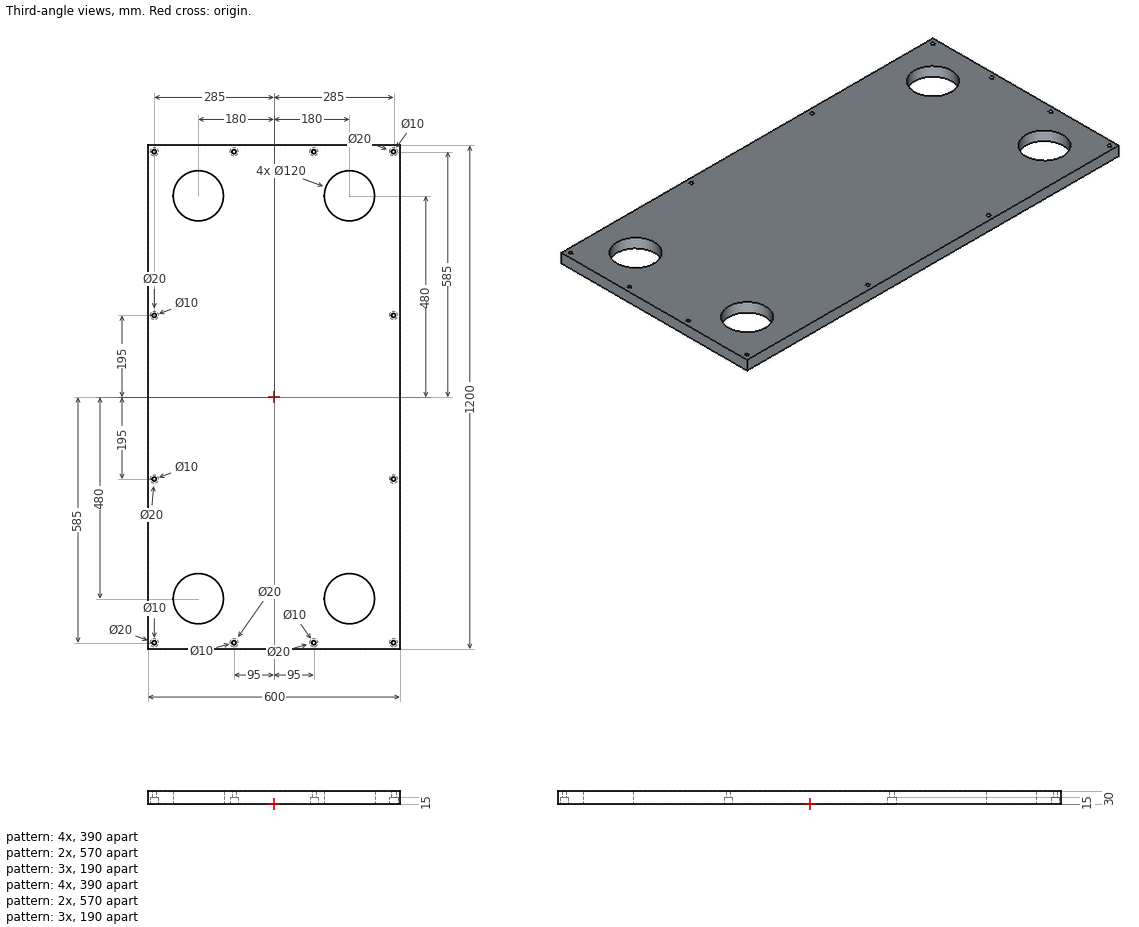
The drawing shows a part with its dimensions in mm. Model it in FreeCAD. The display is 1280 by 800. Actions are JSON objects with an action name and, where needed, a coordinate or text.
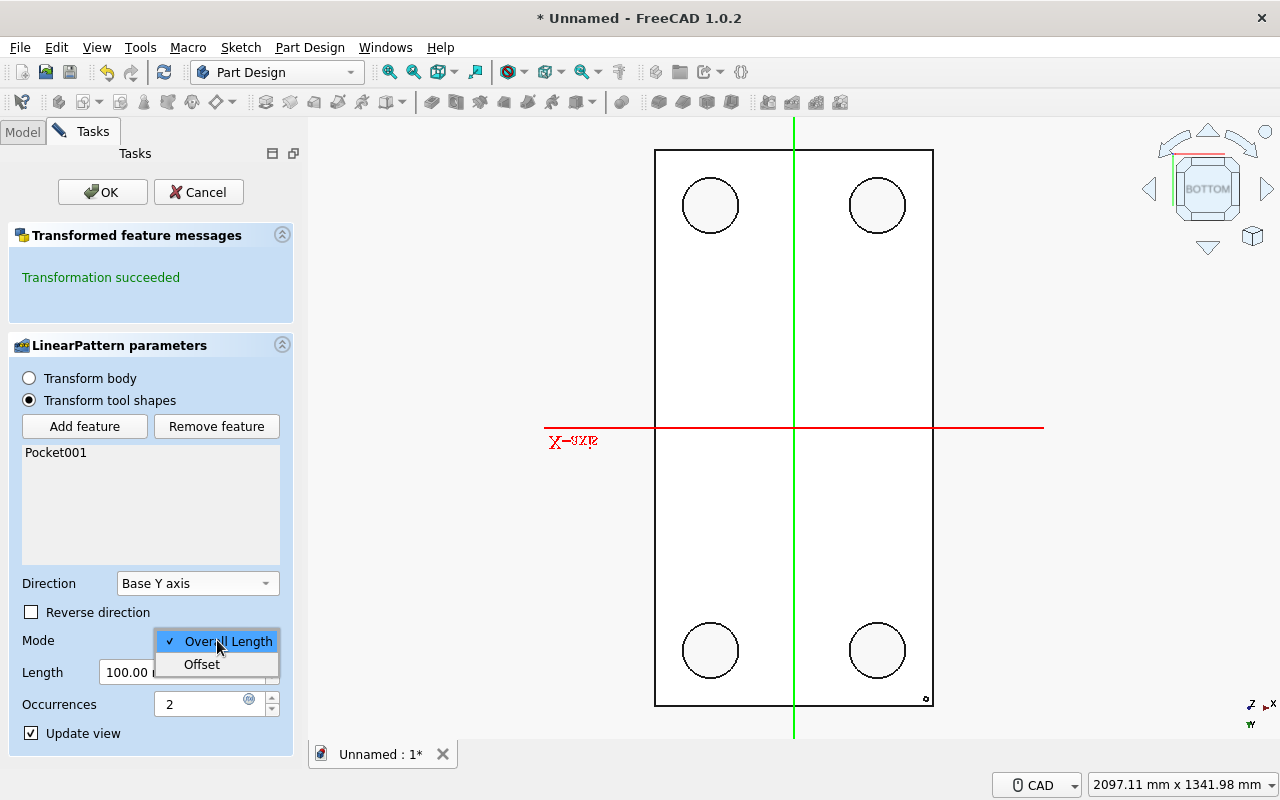
{"action": "left_click", "coordinate": [216, 664]}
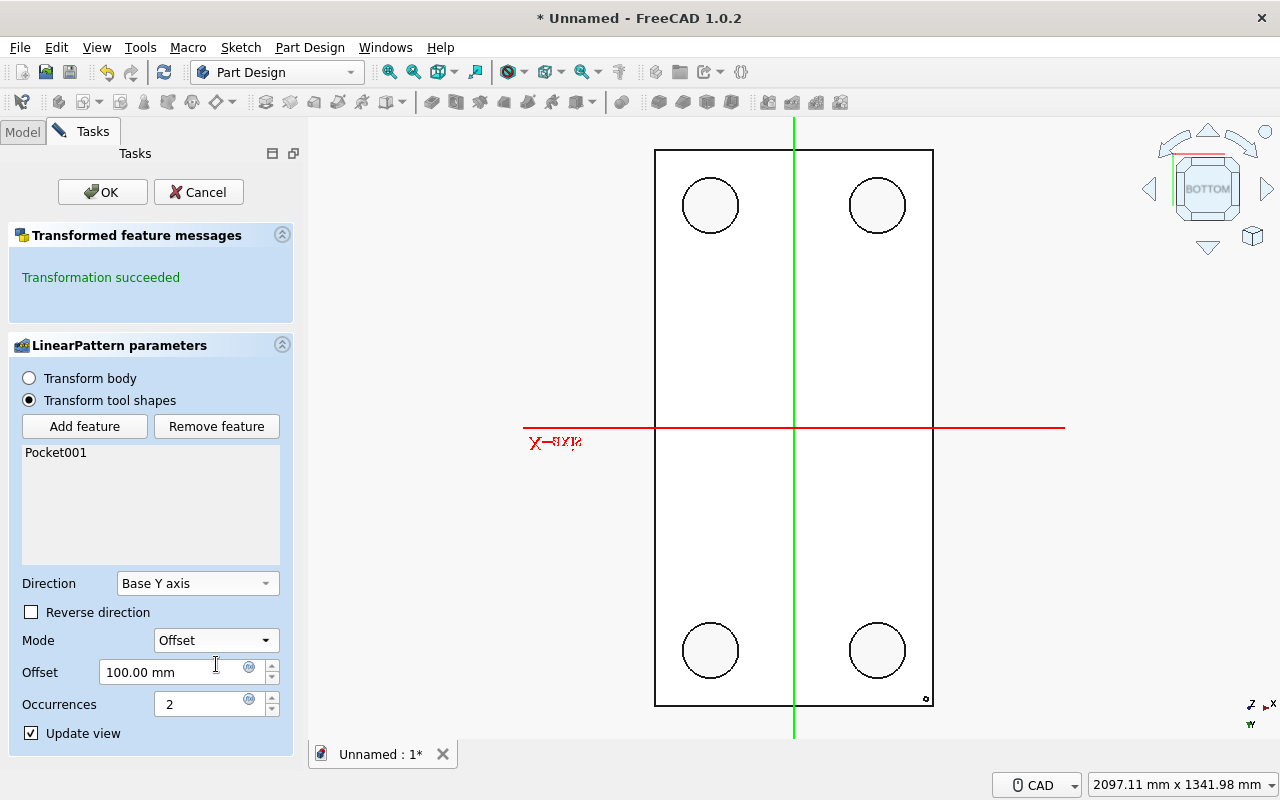
{"action": "triple_click", "coordinate": [182, 672]}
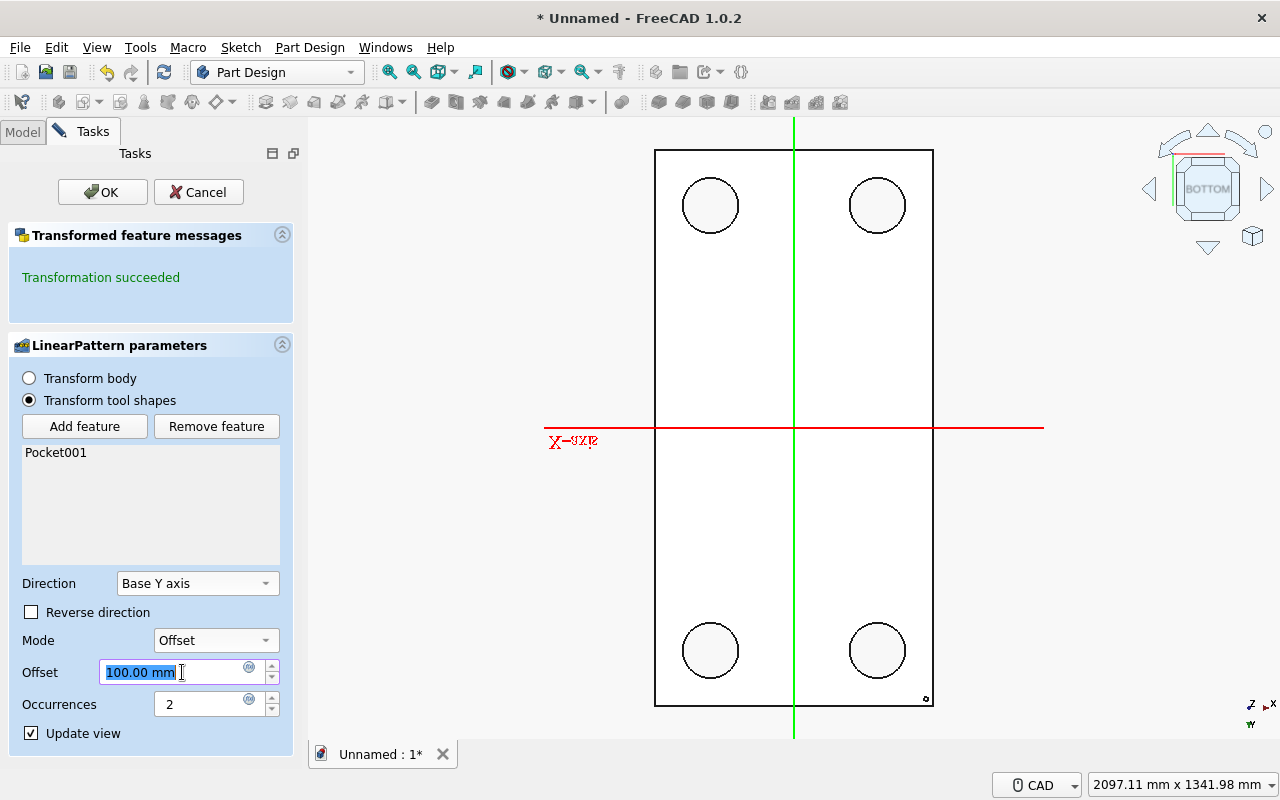
{"action": "type", "text": "390"}
{"action": "key", "text": "Tab"}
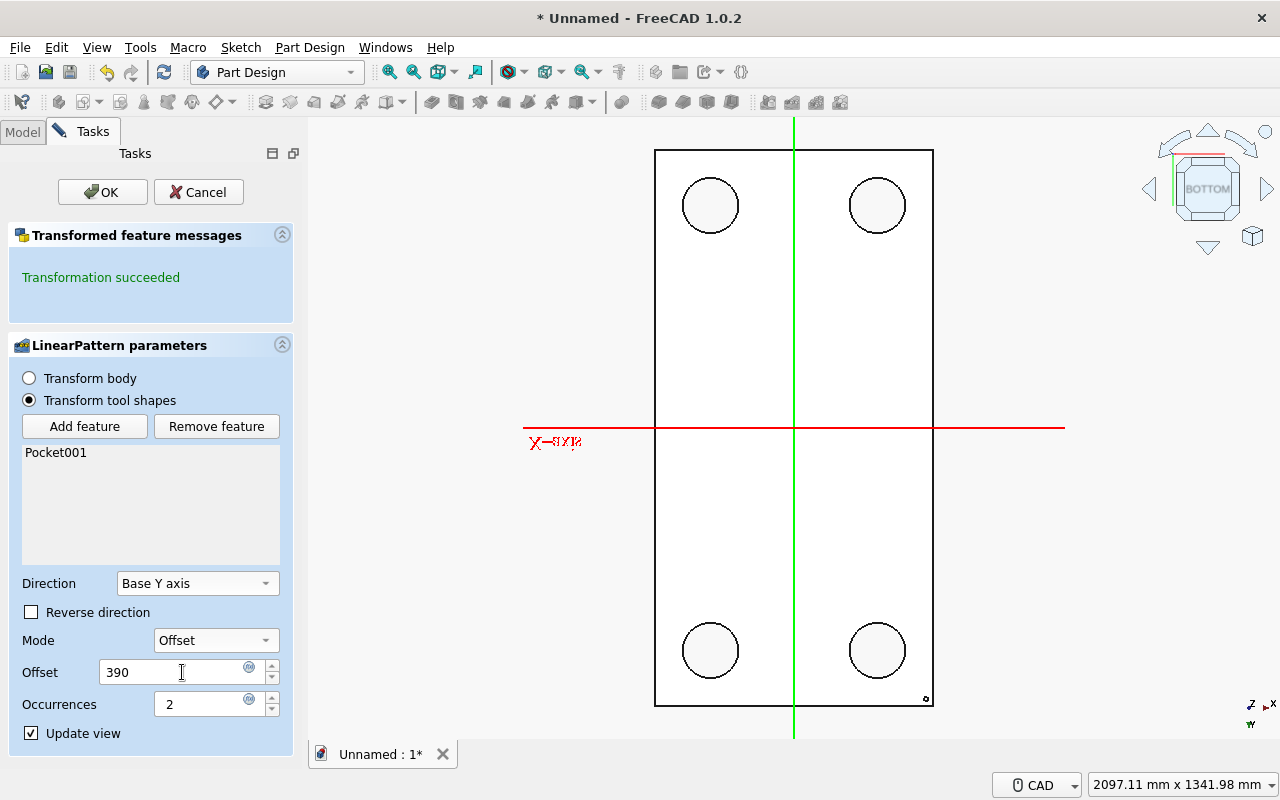
{"action": "triple_click", "coordinate": [209, 704]}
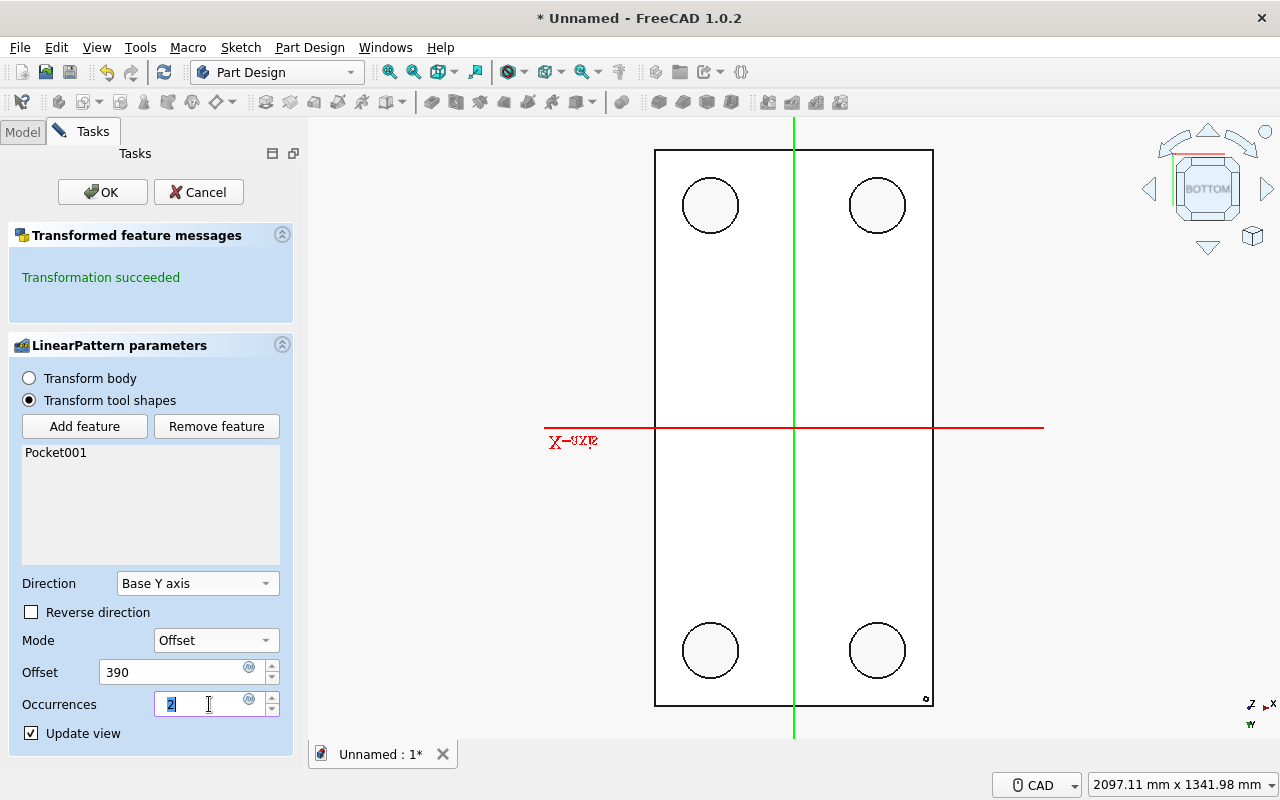
{"action": "type", "text": "4"}
{"action": "key", "text": "Tab"}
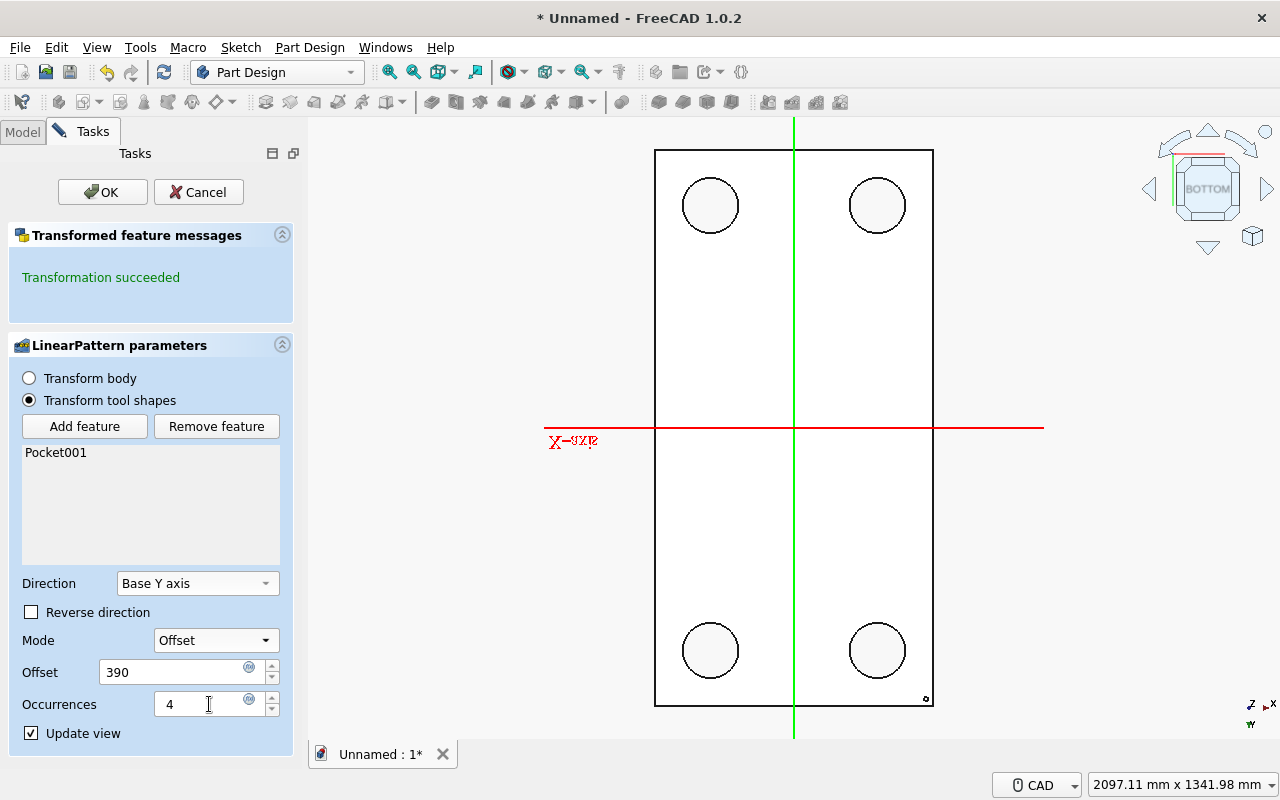
{"action": "left_click", "coordinate": [30, 612]}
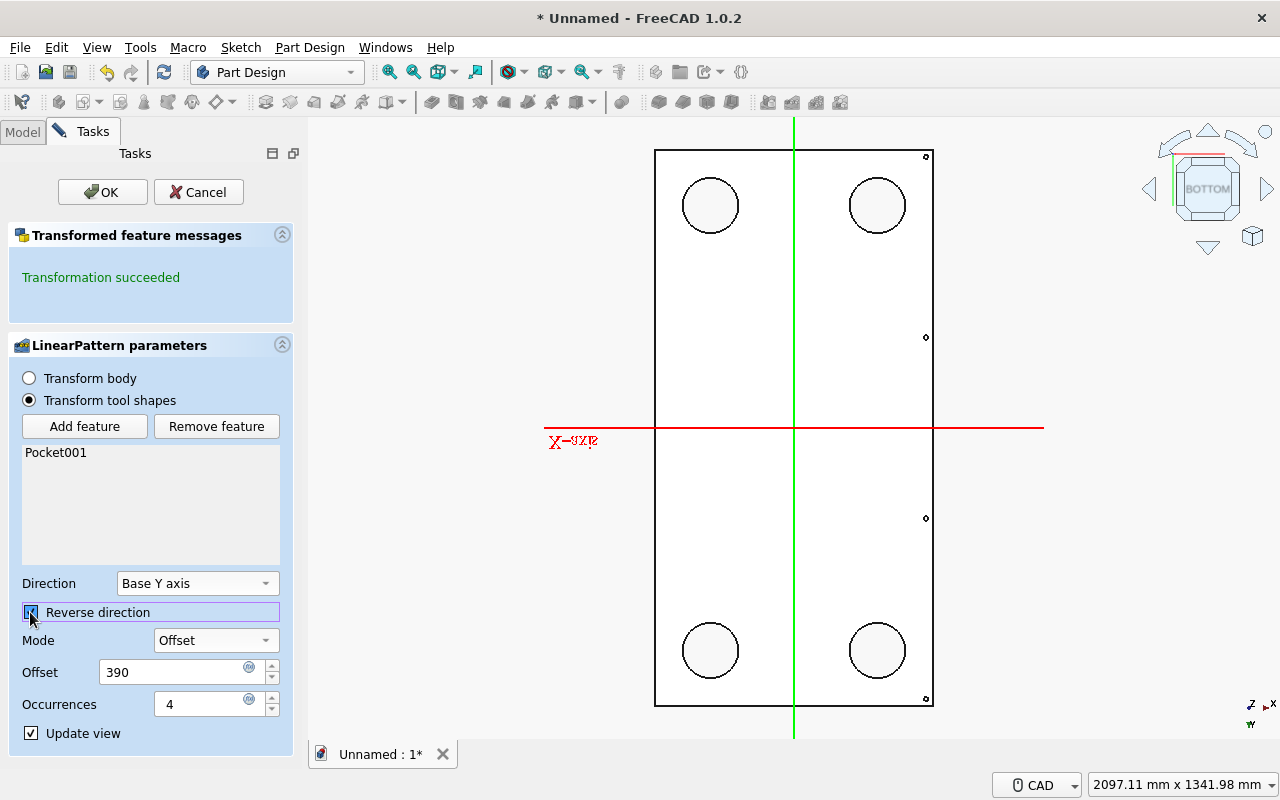
{"action": "left_click", "coordinate": [103, 192]}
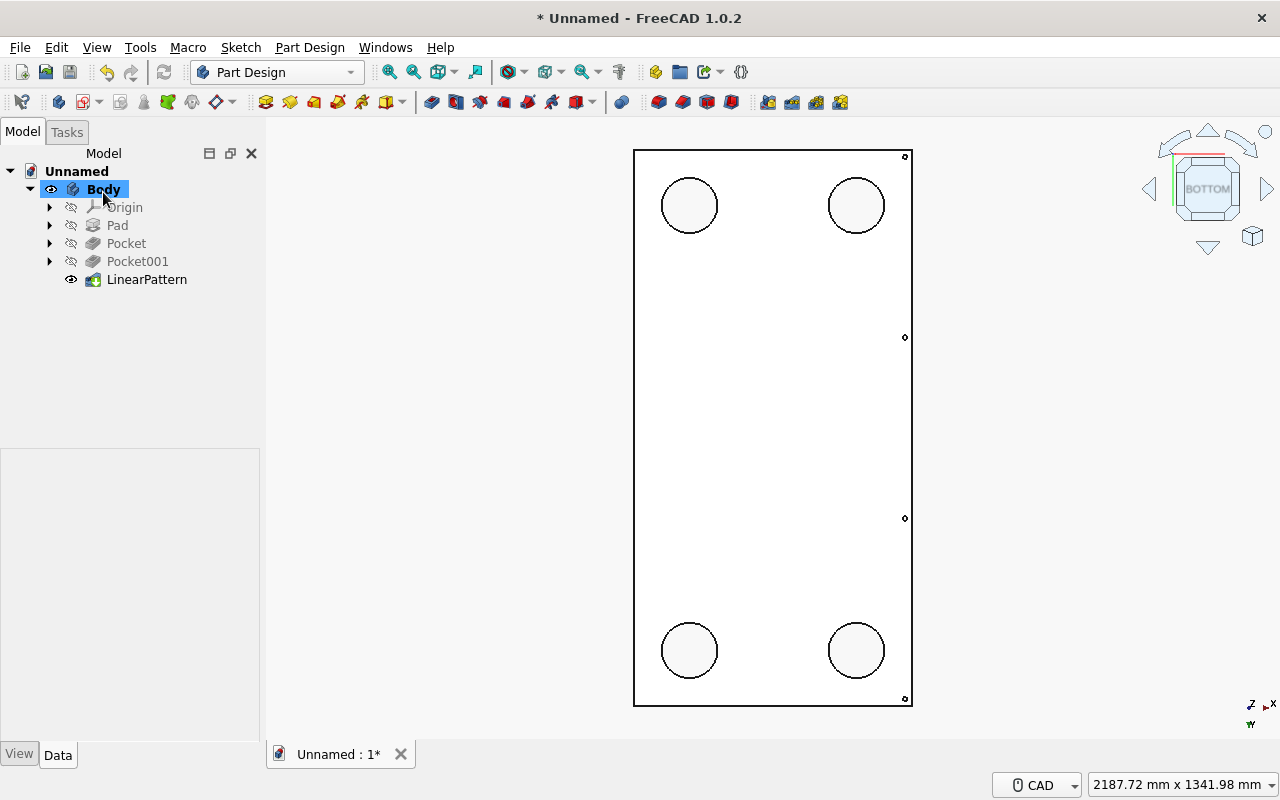
{"action": "left_click", "coordinate": [116, 261]}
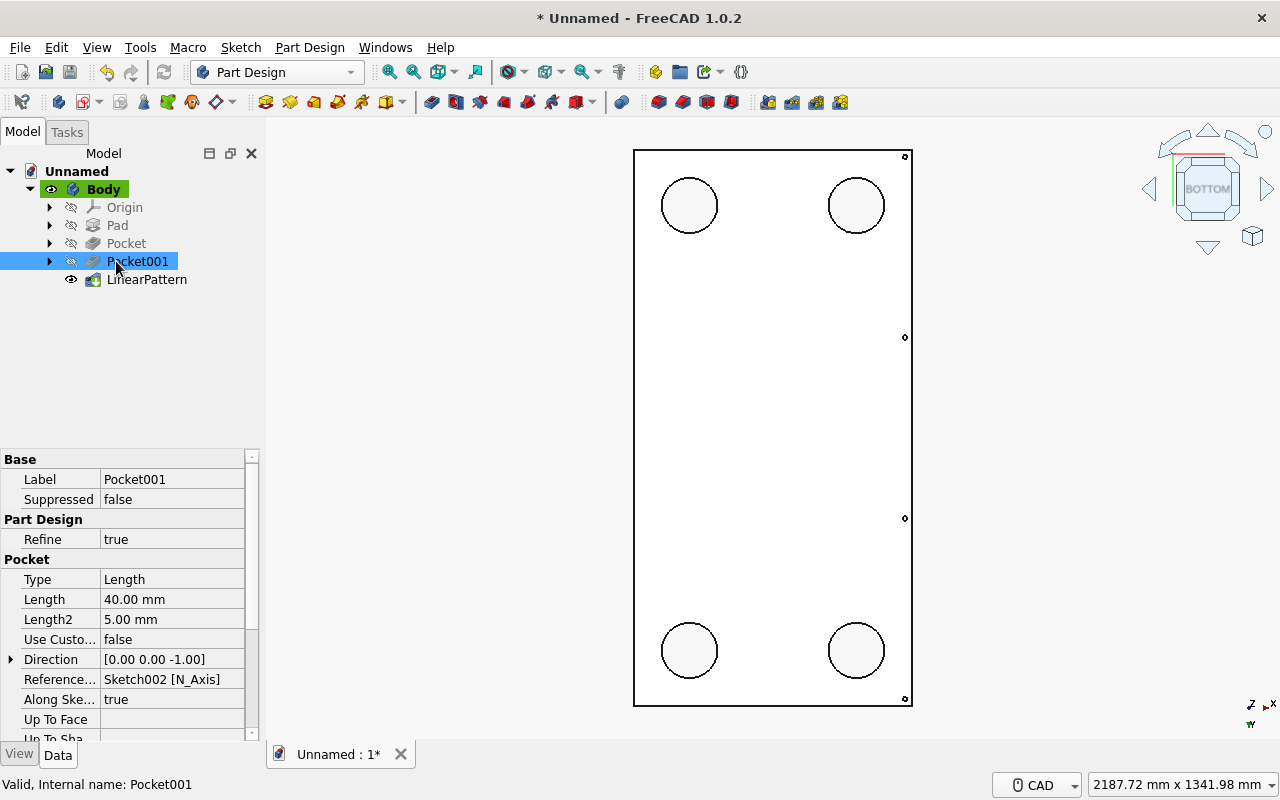
{"action": "left_click", "coordinate": [792, 102]}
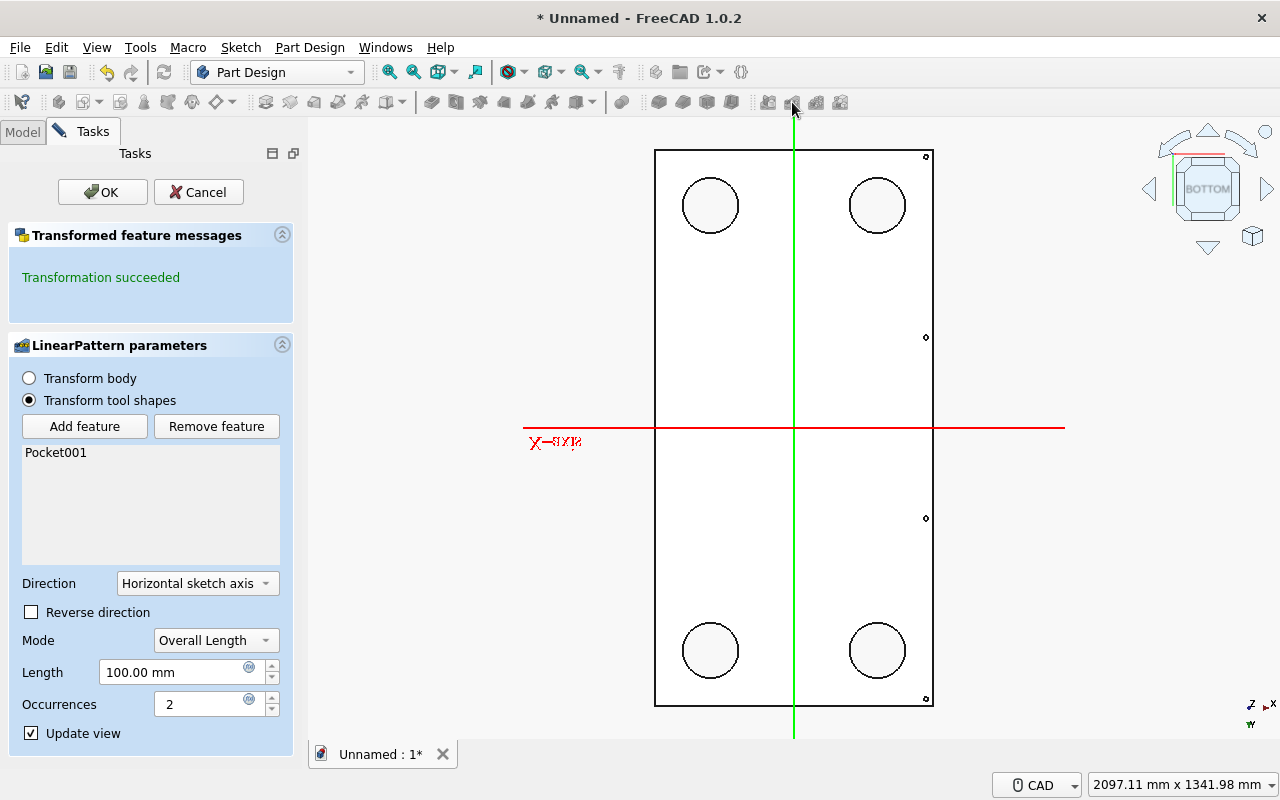
{"action": "left_click", "coordinate": [198, 584]}